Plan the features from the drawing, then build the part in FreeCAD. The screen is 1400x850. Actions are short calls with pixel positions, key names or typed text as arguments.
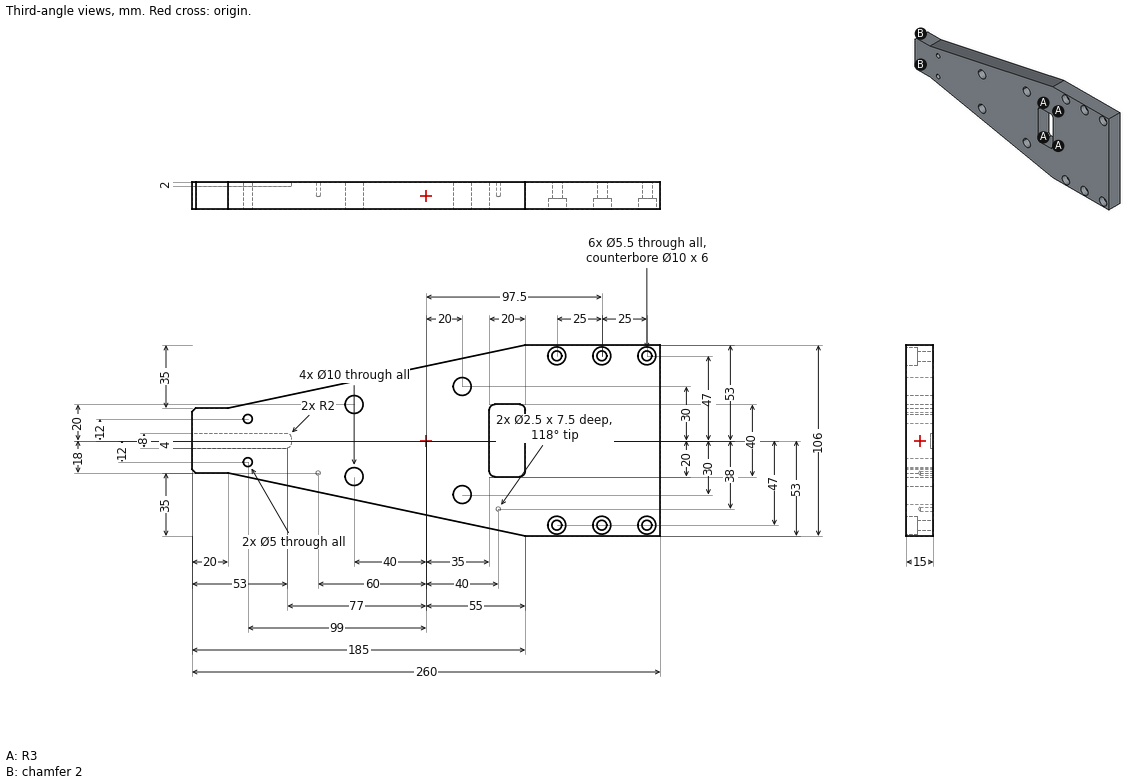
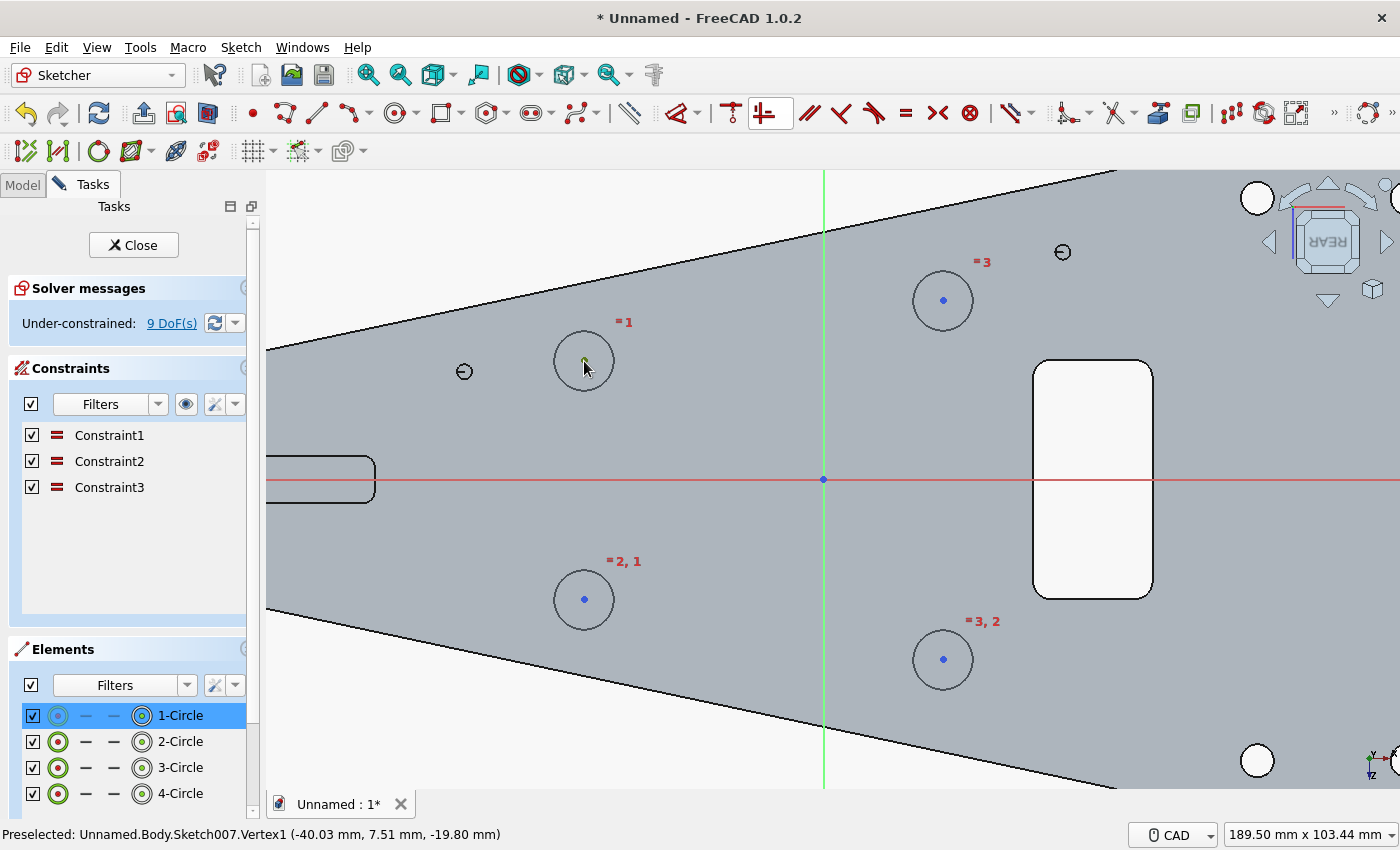
click(584, 600)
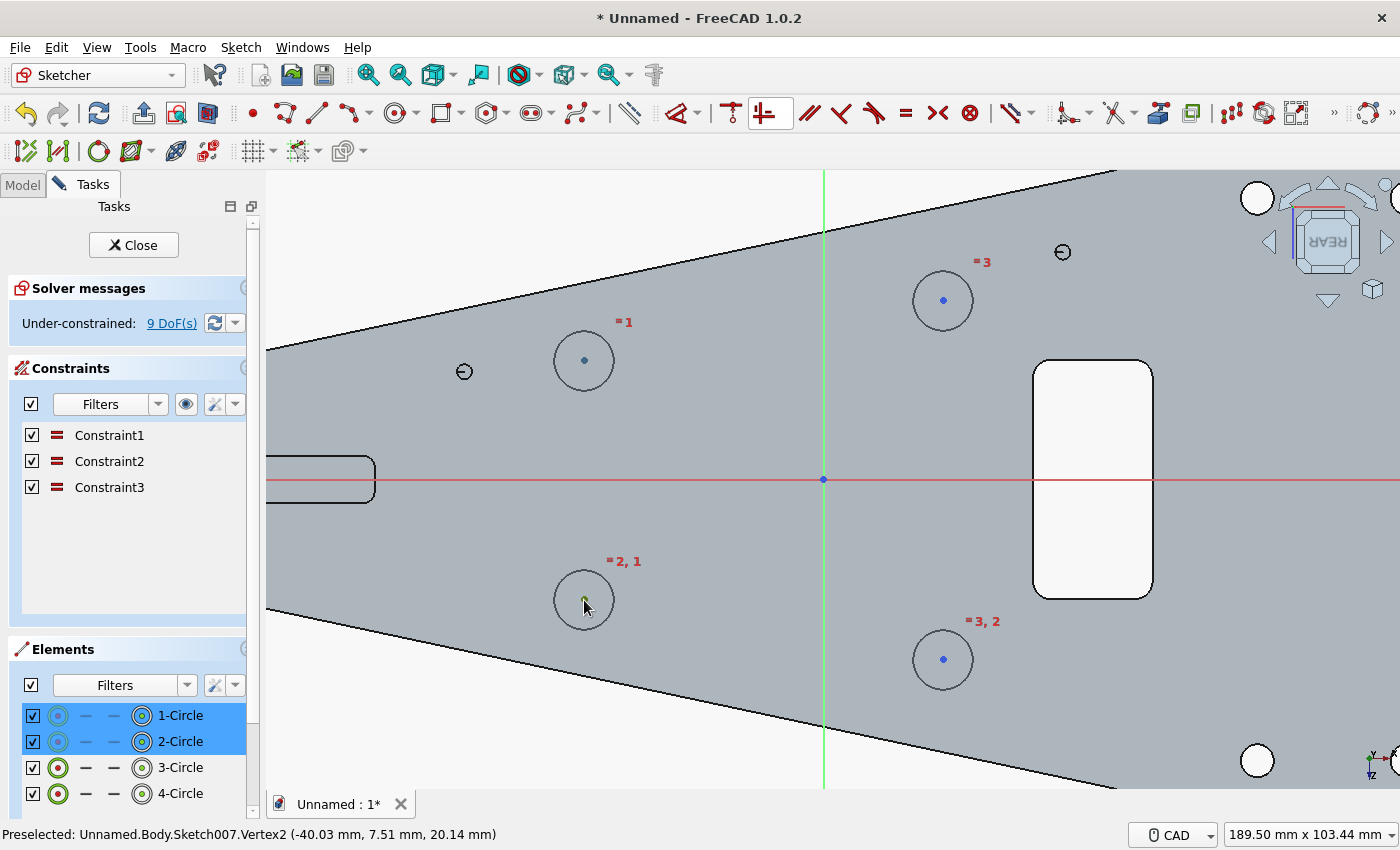
key(v)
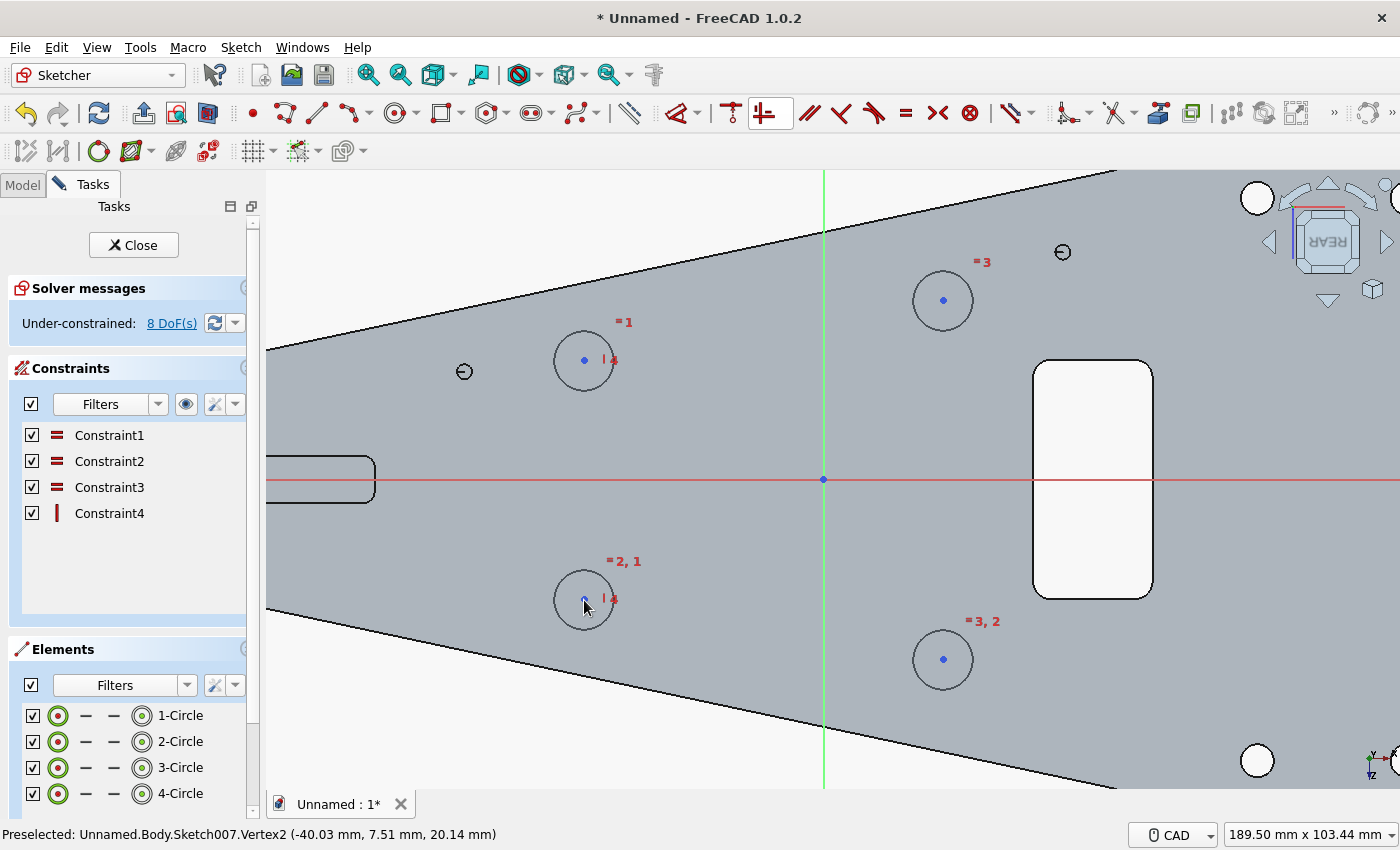
click(943, 660)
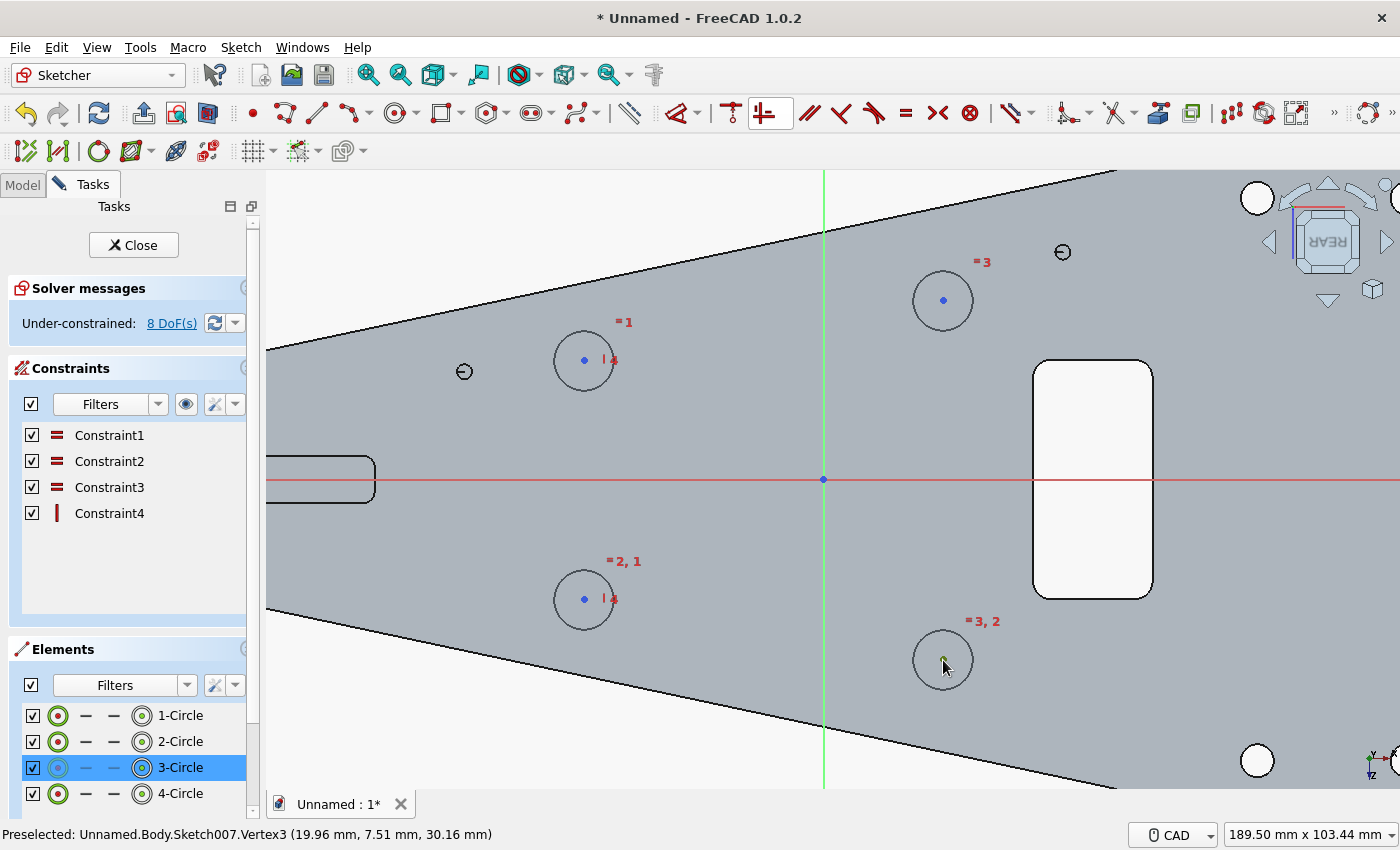
click(943, 301)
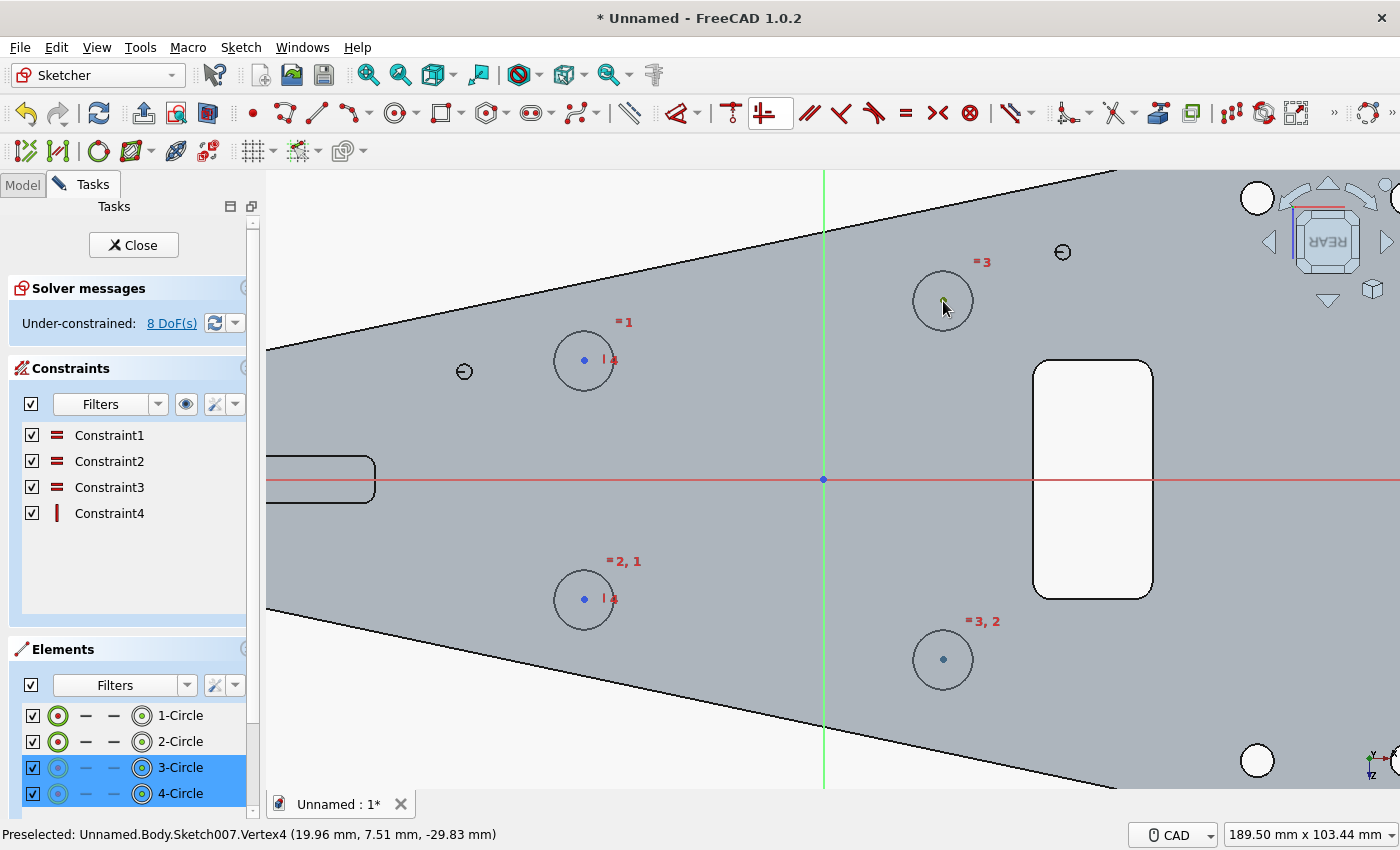
key(v)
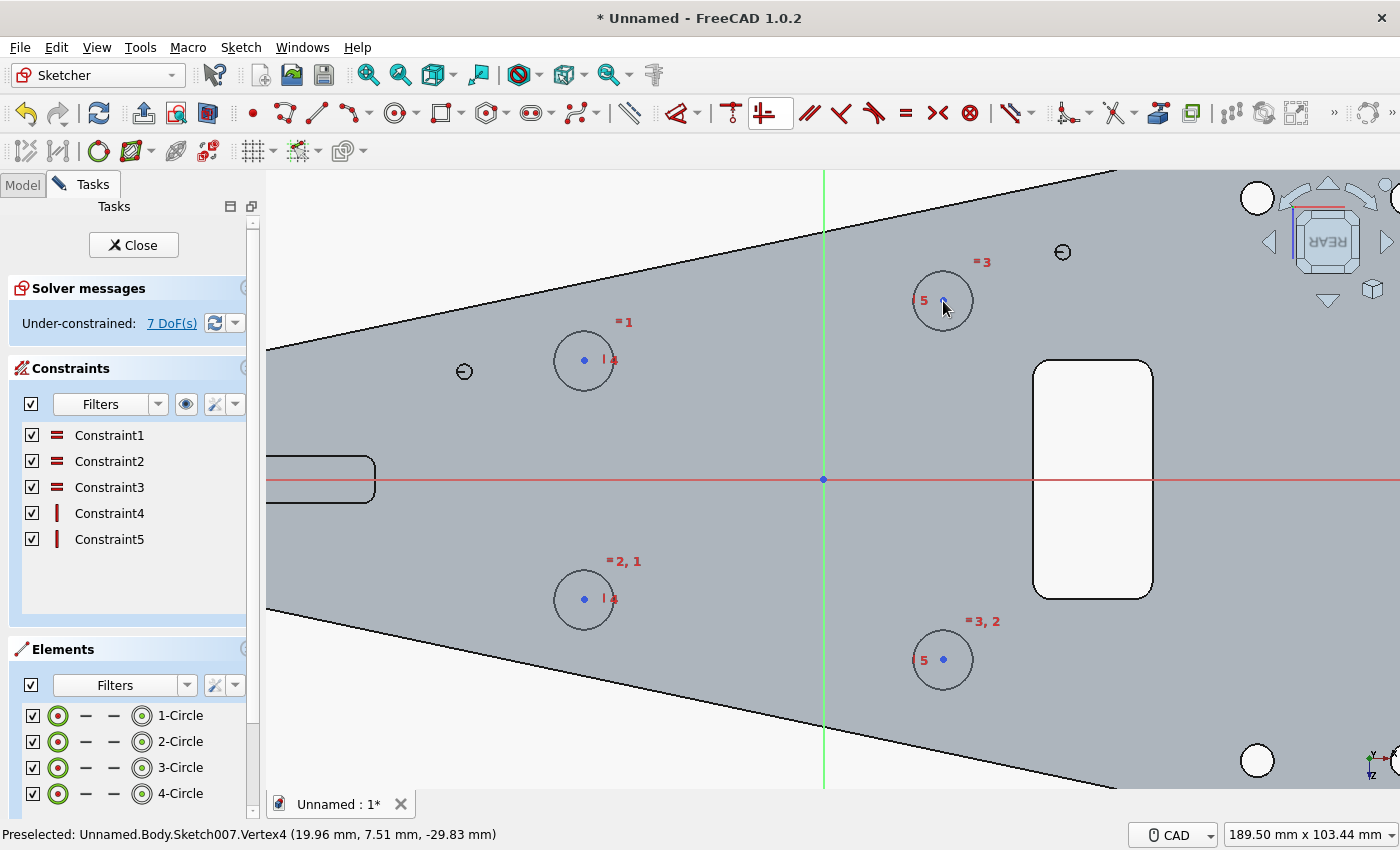
key(d)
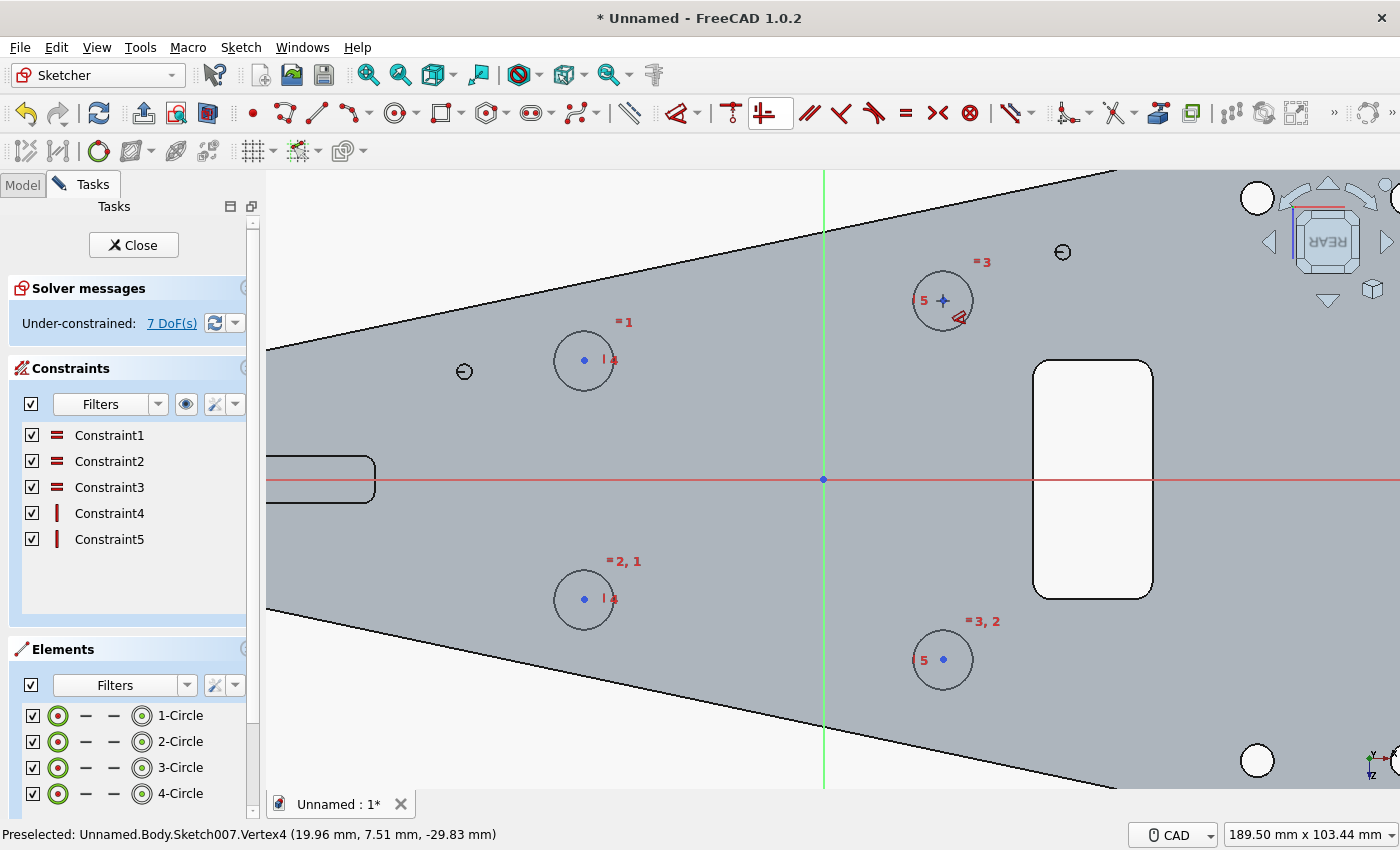
click(605, 340)
click(628, 317)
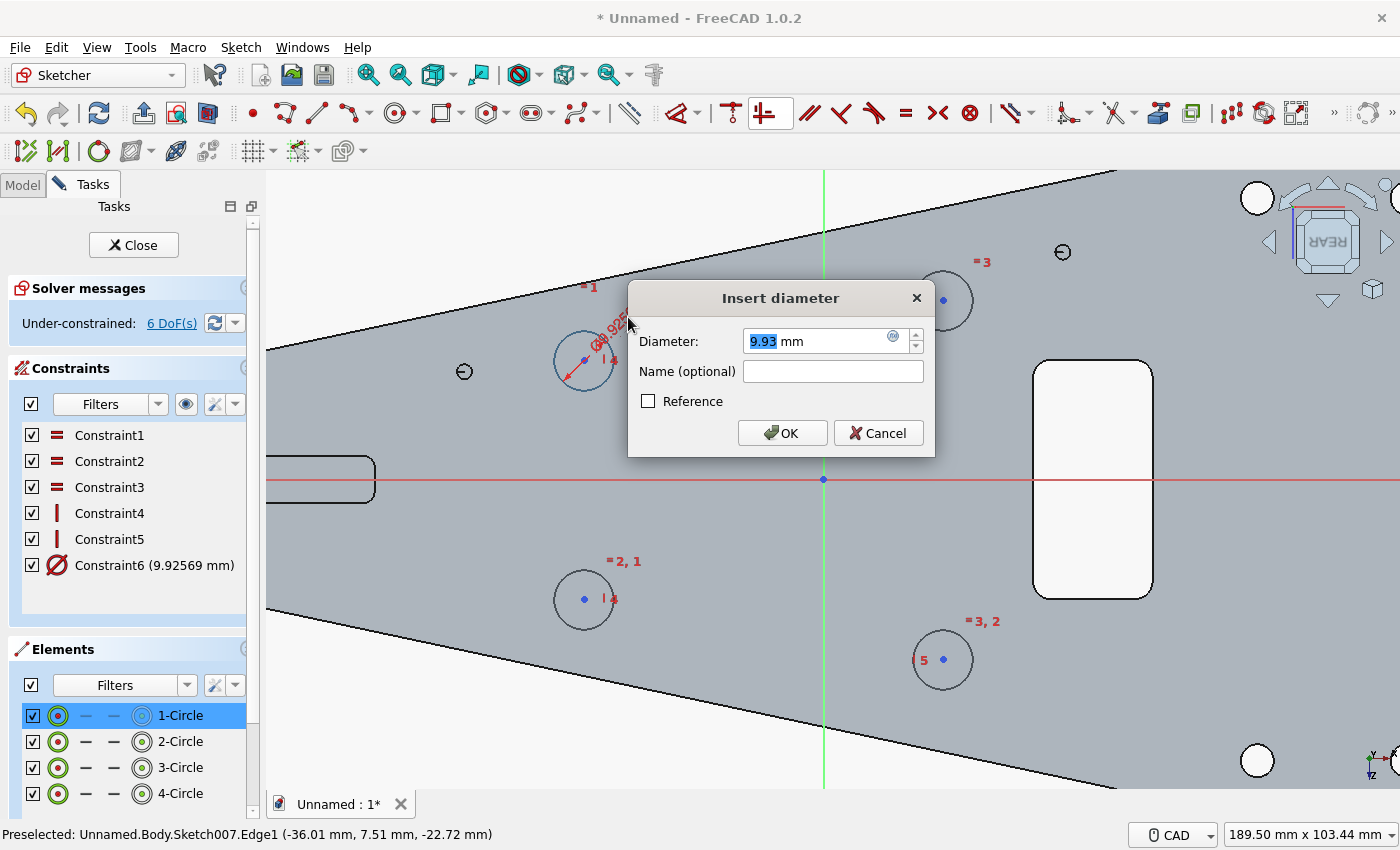
text(10)
key(Return)